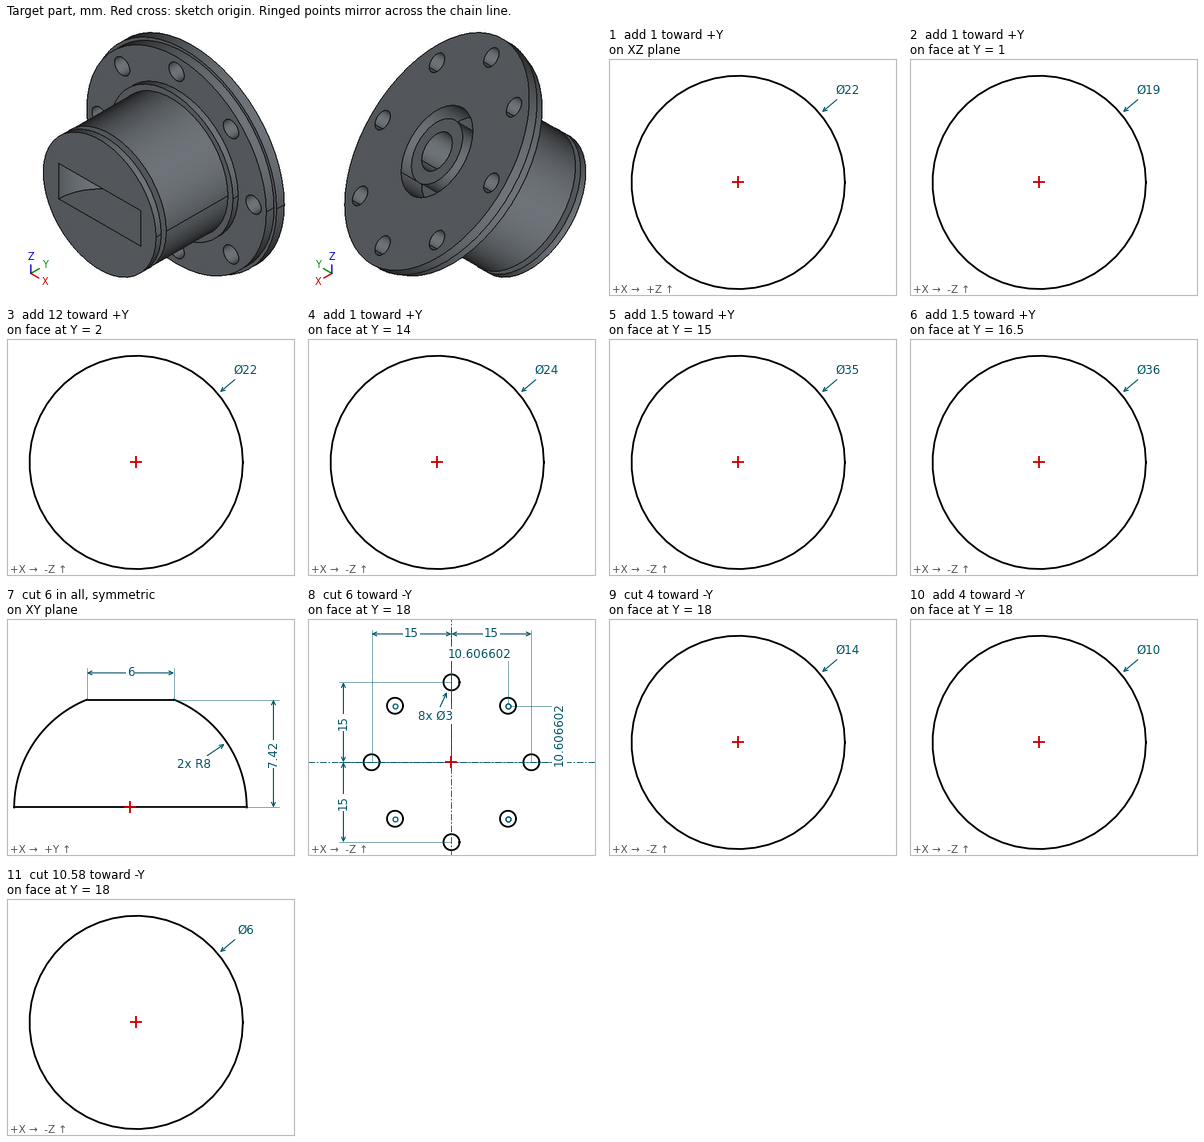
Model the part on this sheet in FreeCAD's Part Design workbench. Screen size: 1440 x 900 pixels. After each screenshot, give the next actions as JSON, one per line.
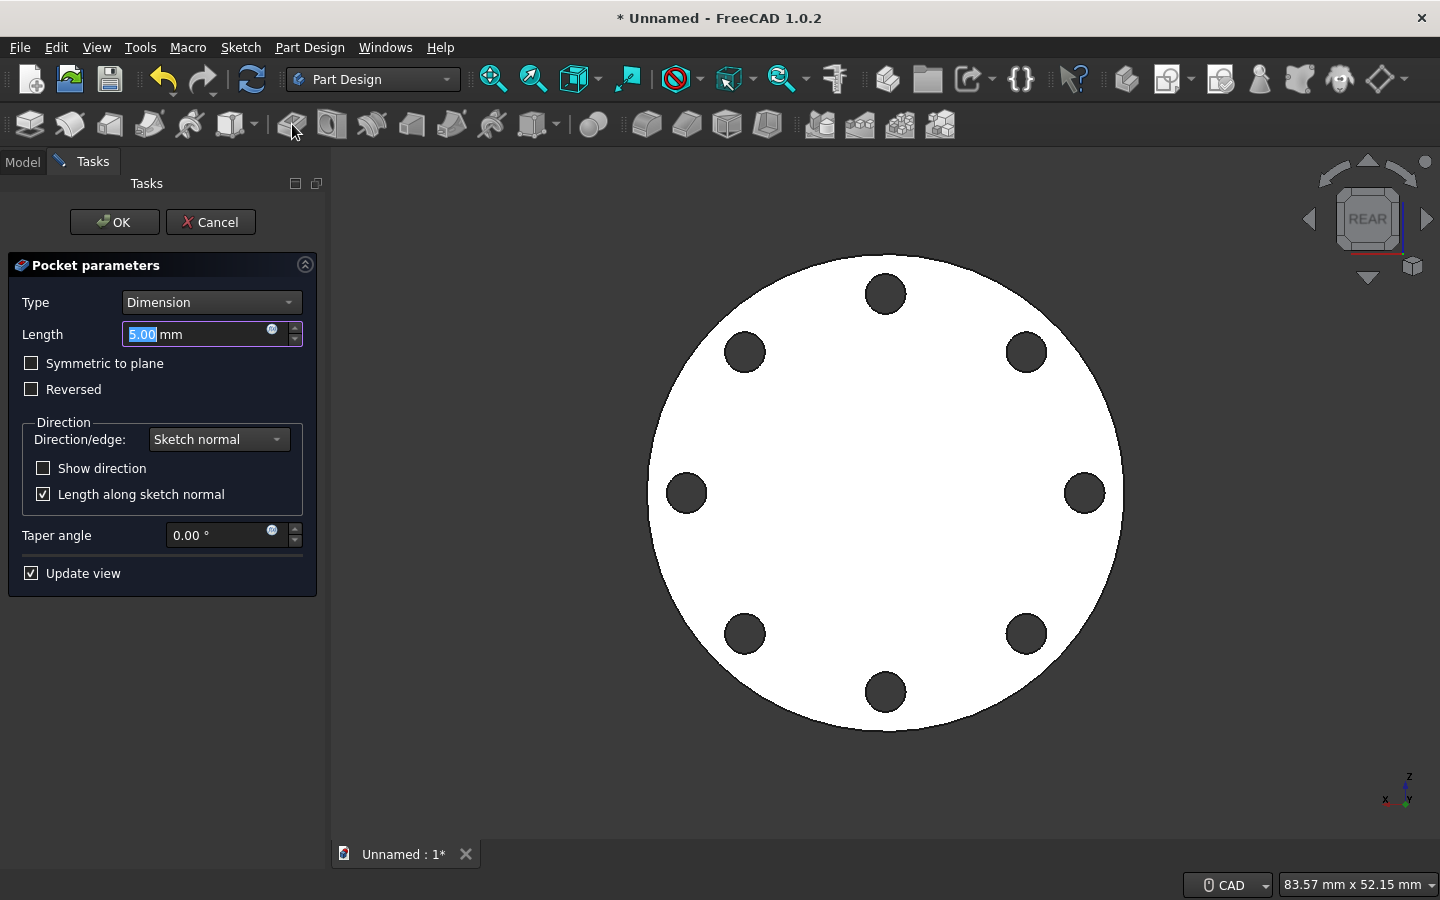
{"action": "type", "text": "6"}
{"action": "key", "text": "Tab"}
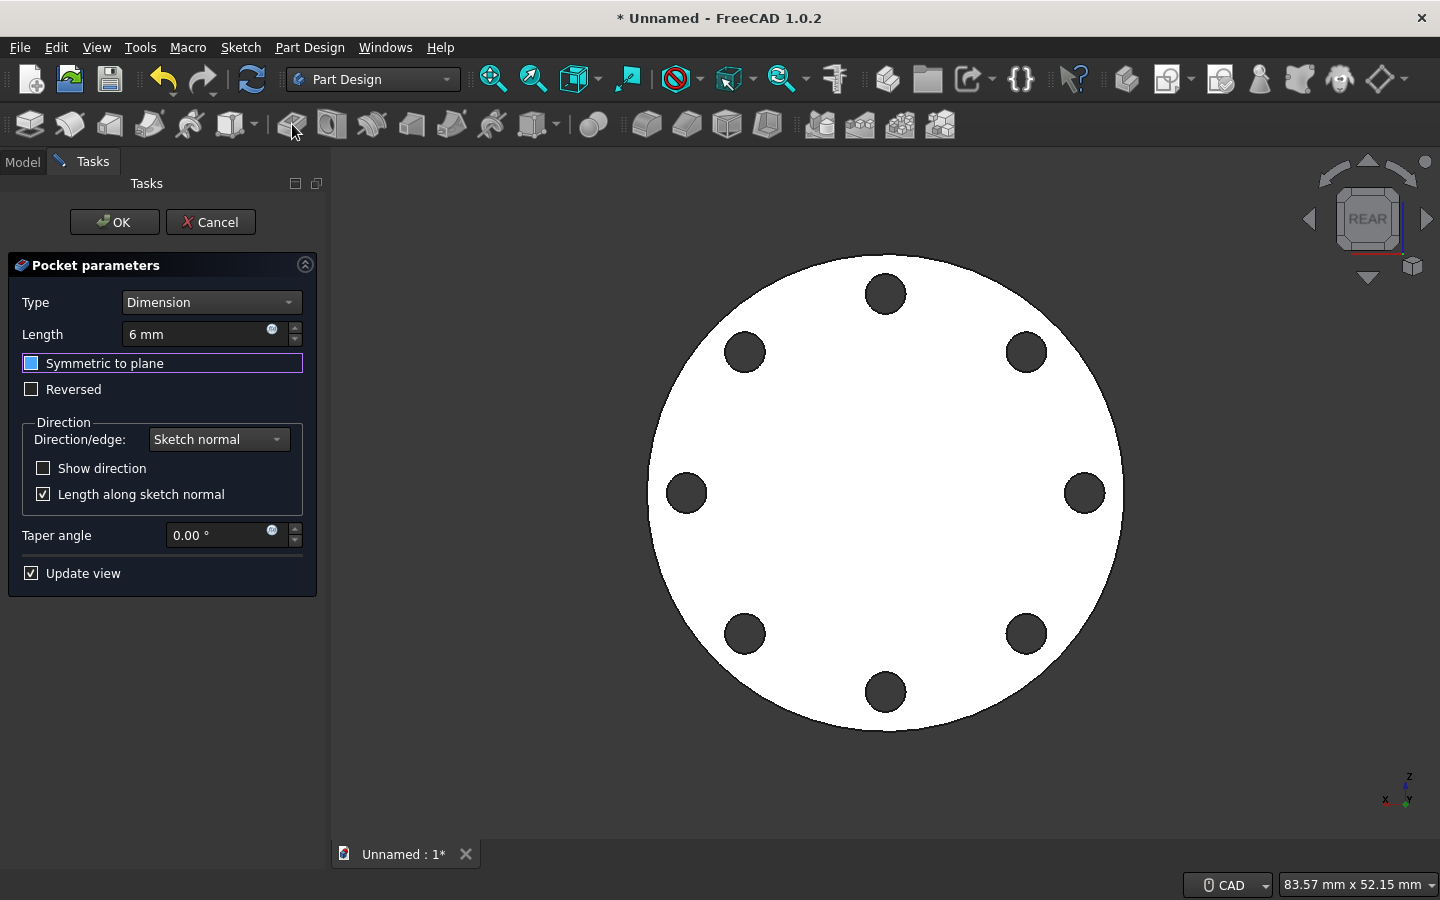
{"action": "left_click", "coordinate": [115, 222]}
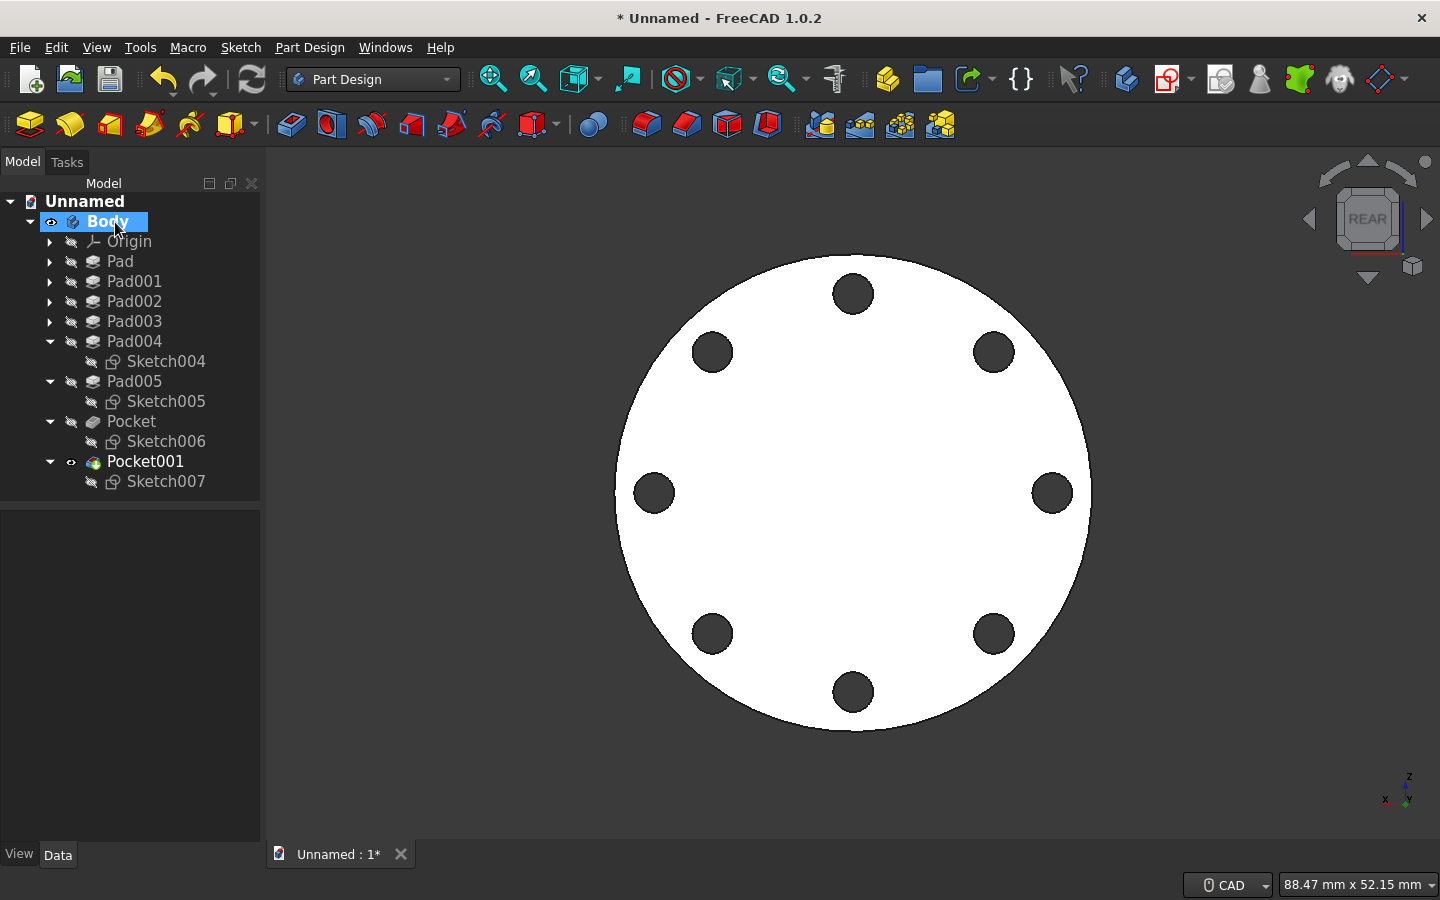
{"action": "left_click", "coordinate": [853, 492]}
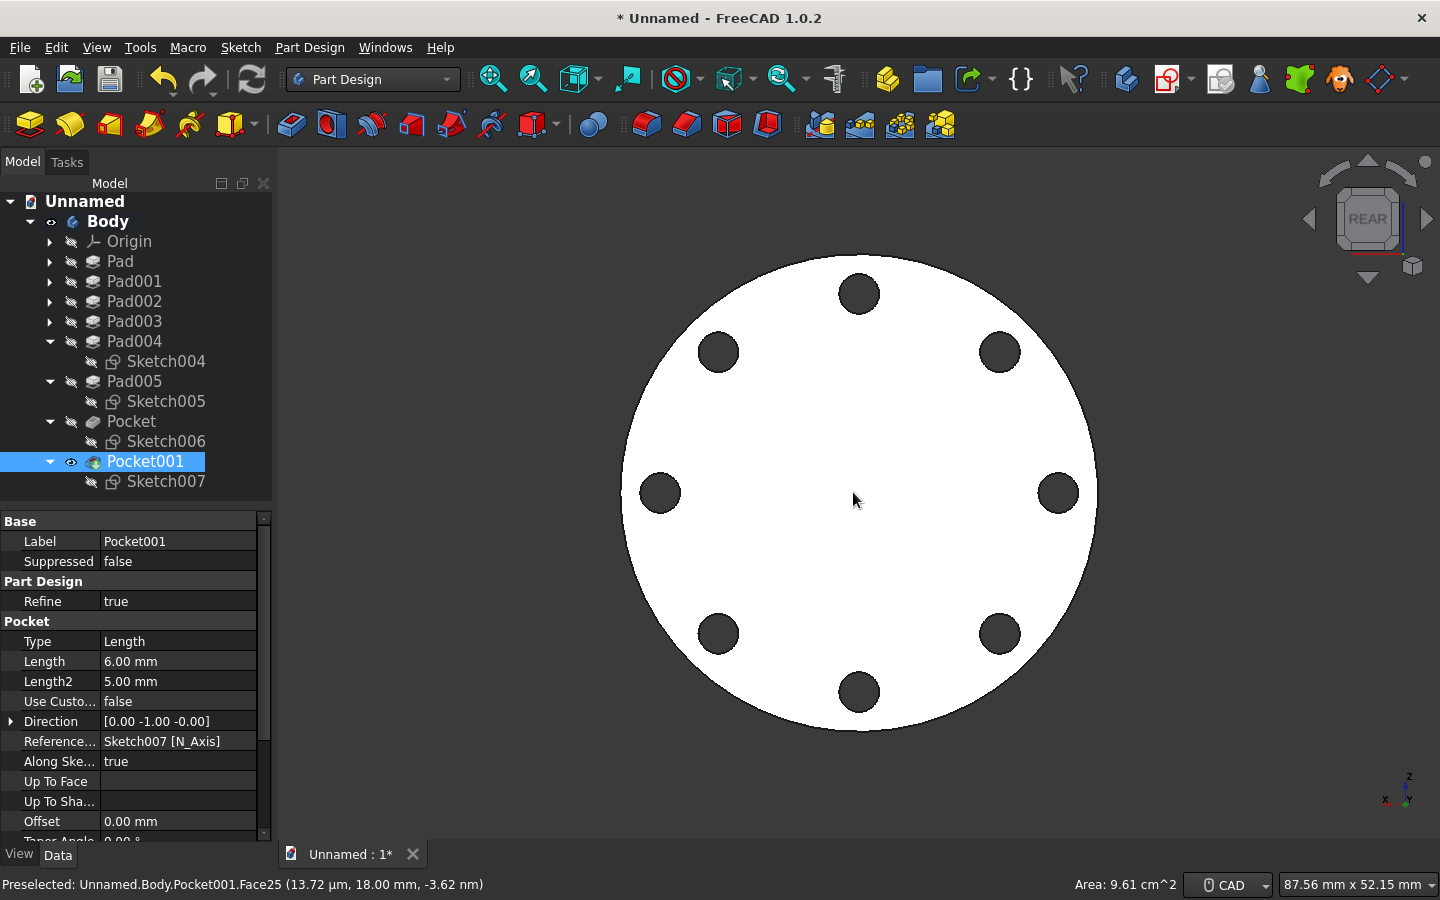
{"action": "left_click", "coordinate": [1168, 80]}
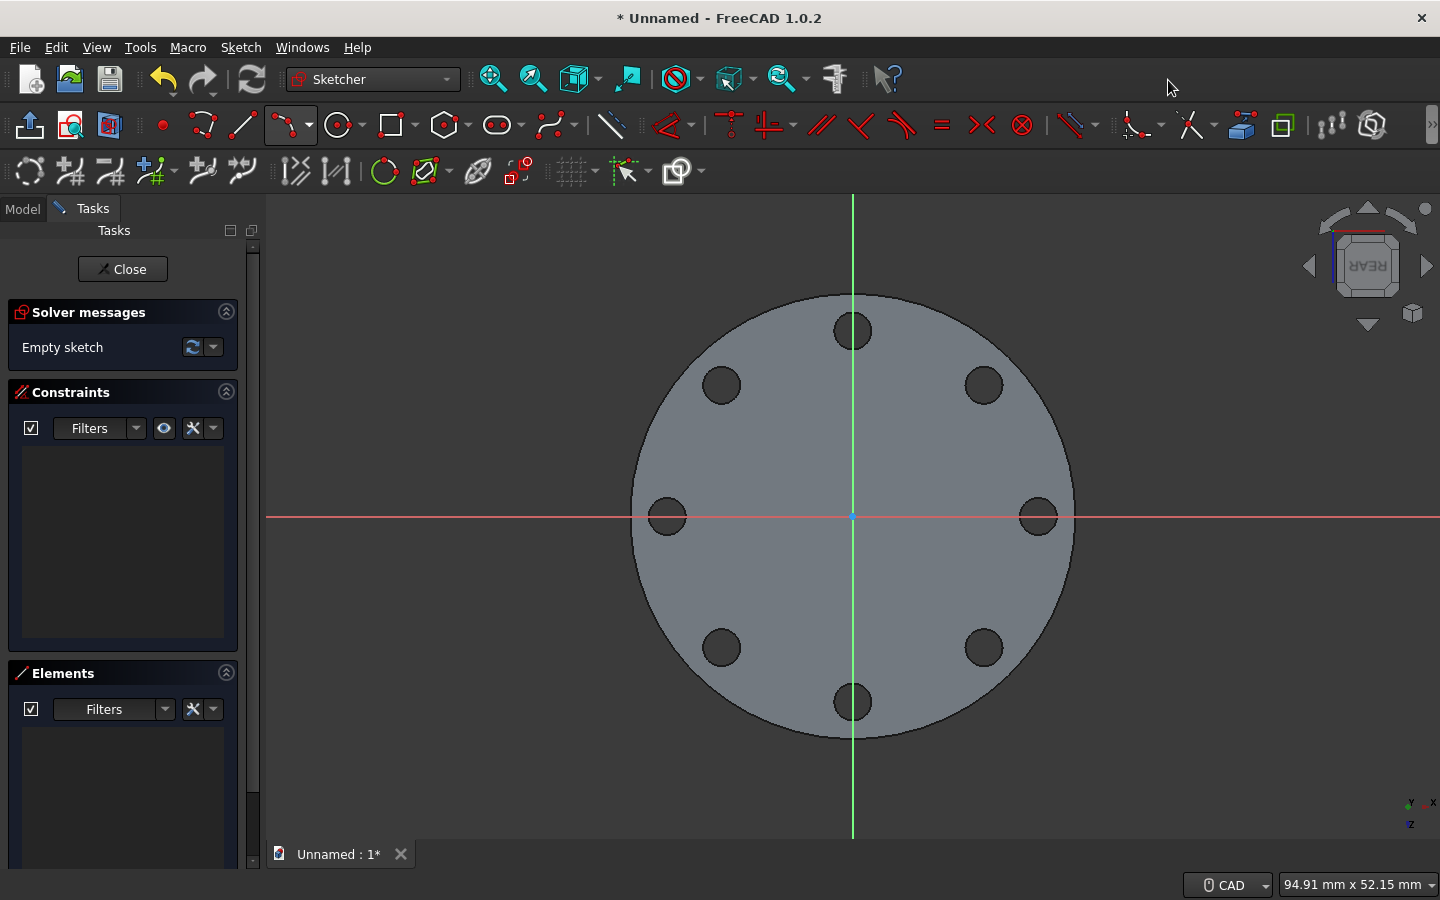
{"action": "scroll", "coordinate": [909, 516], "scroll_direction": "up", "scroll_amount": 4}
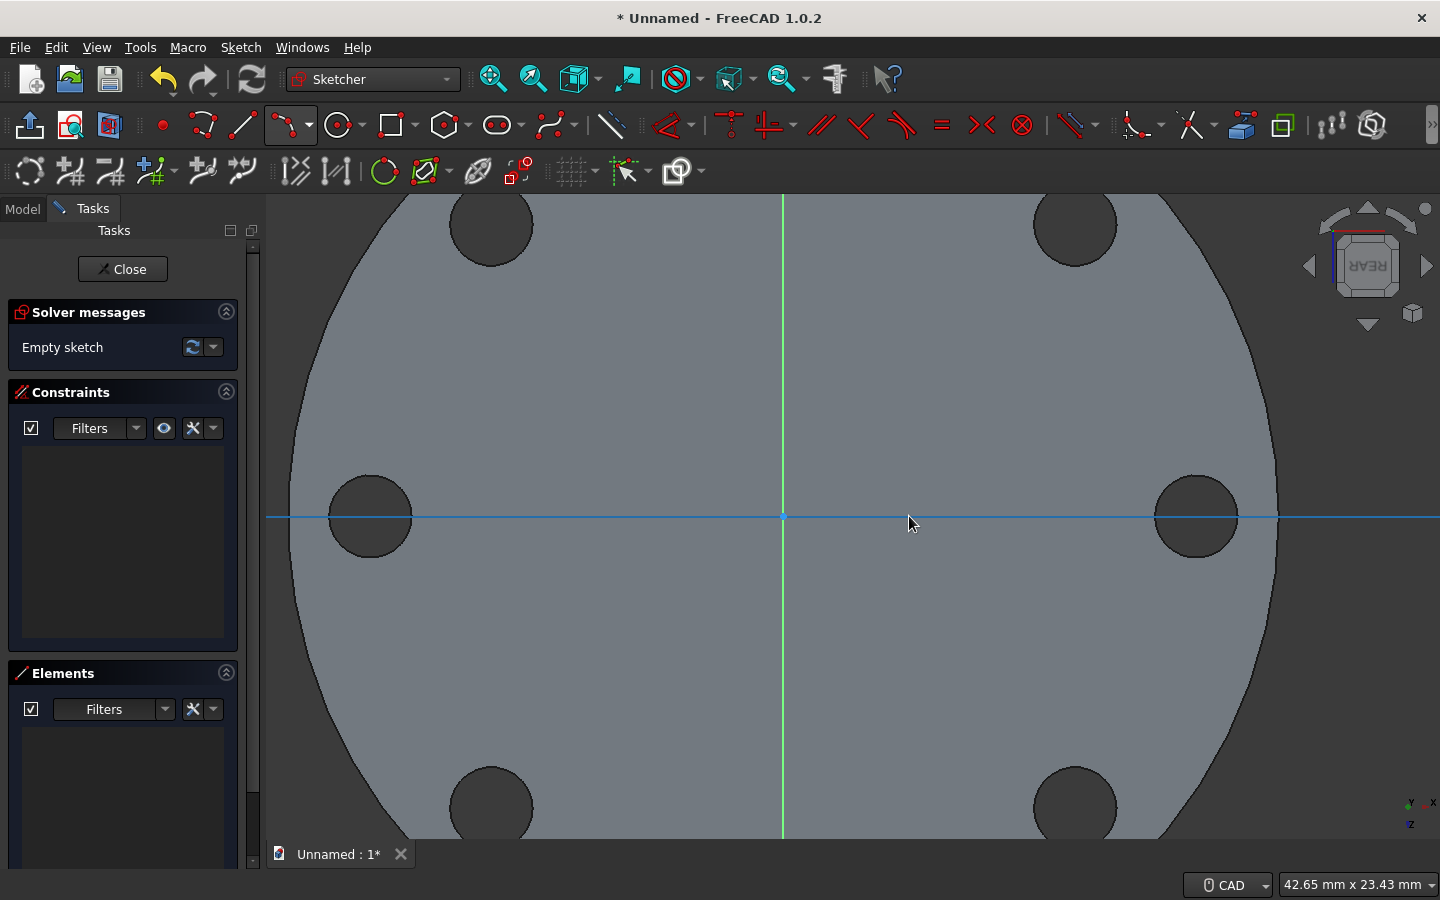
{"action": "left_click", "coordinate": [338, 126]}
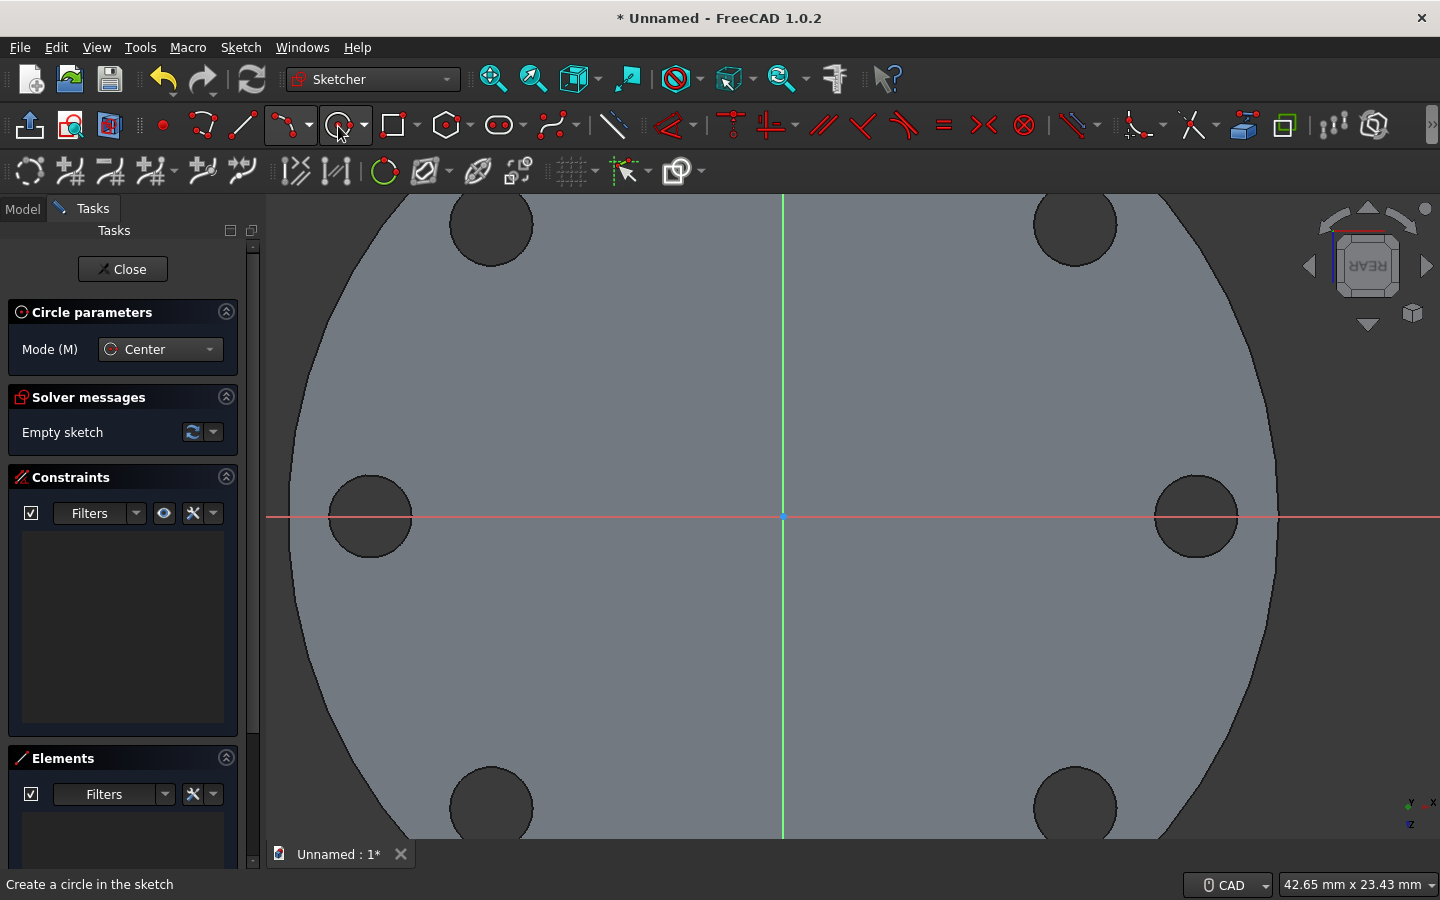
{"action": "left_click", "coordinate": [783, 516]}
{"action": "mouse_move", "coordinate": [920, 380]}